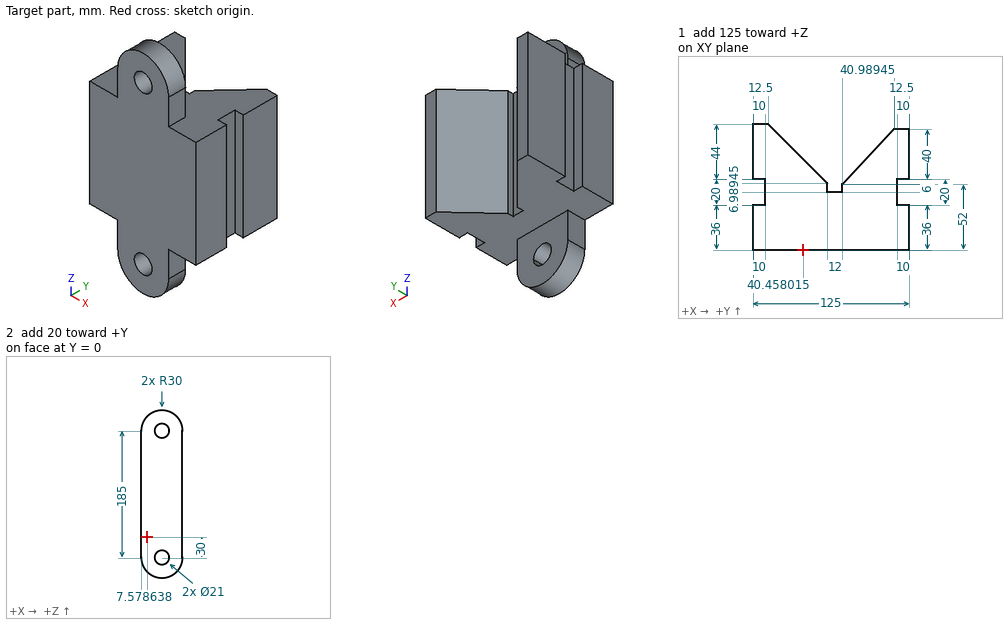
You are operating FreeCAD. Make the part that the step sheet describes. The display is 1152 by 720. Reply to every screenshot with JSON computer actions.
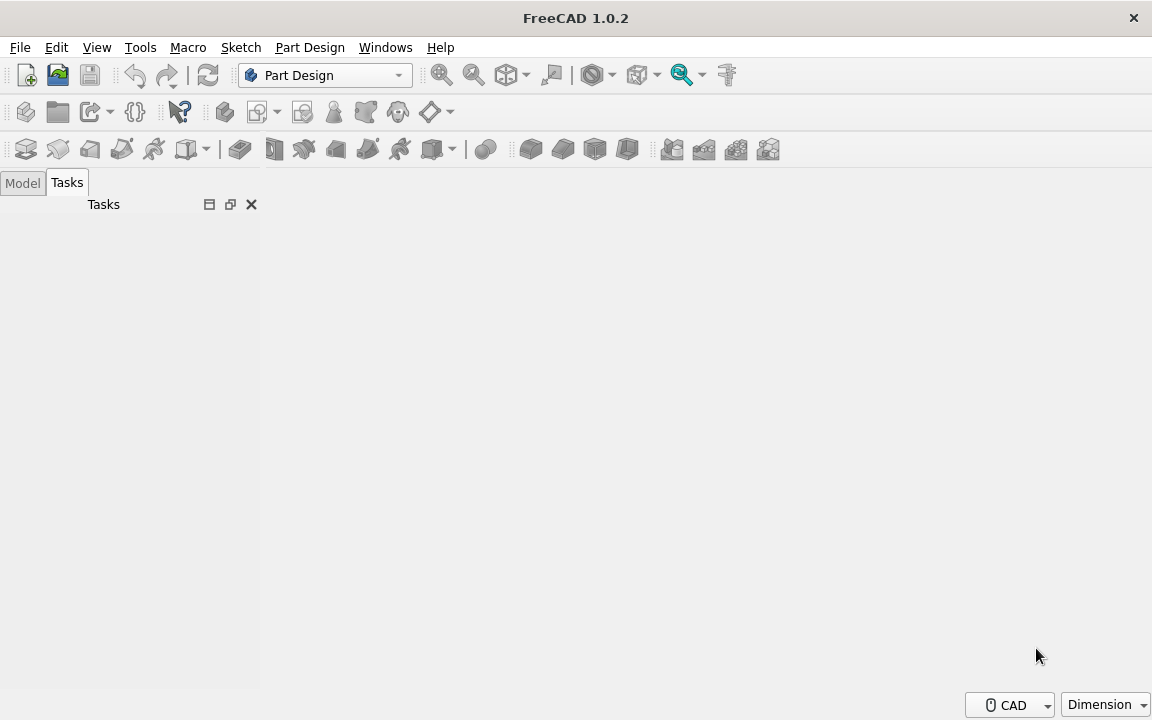
{"action": "key", "text": "ctrl+n"}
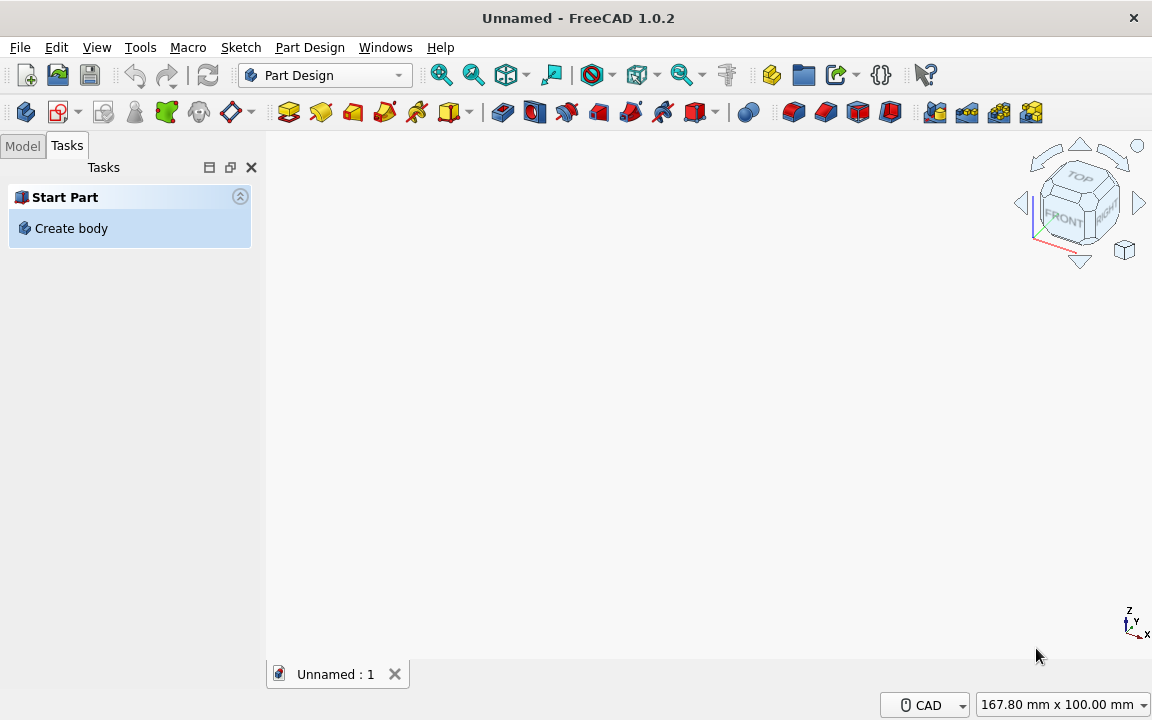
{"action": "left_click", "coordinate": [58, 112]}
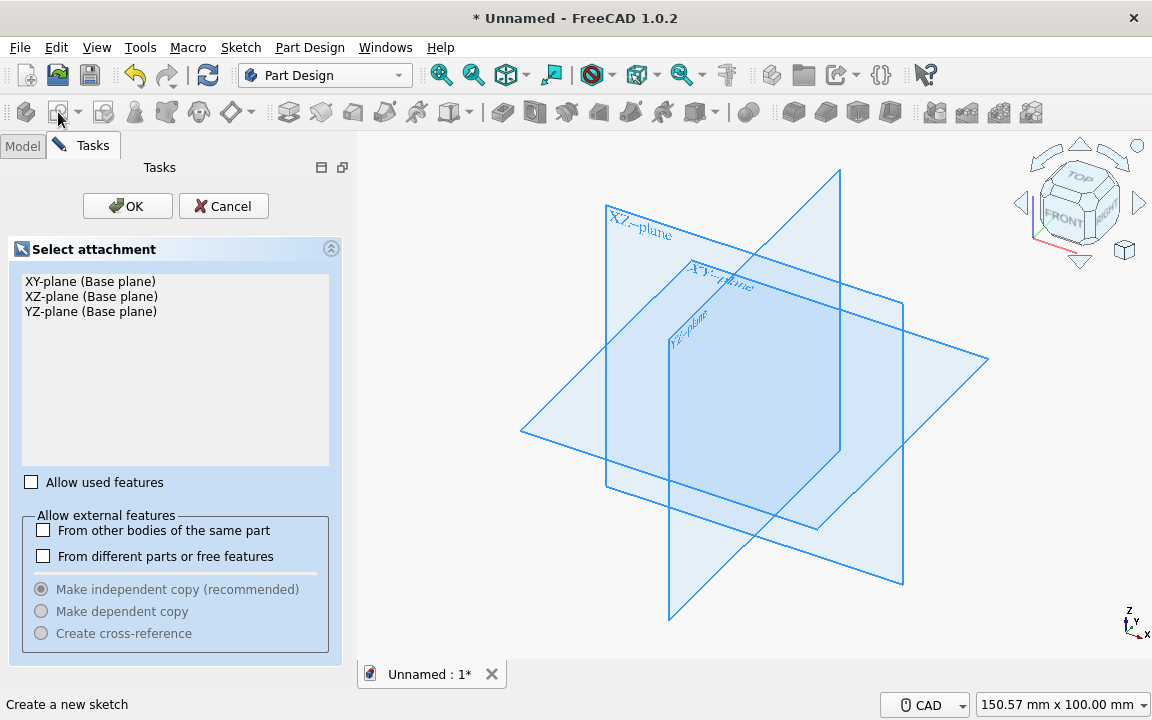
{"action": "left_click", "coordinate": [82, 282]}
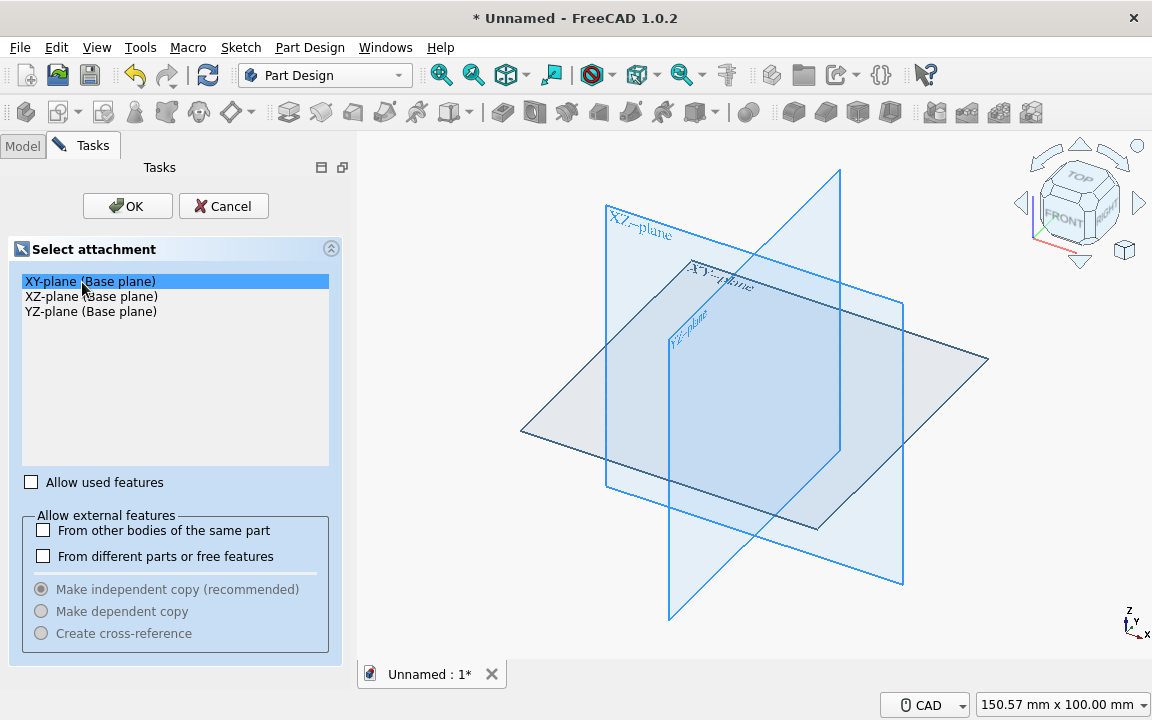
{"action": "left_click", "coordinate": [128, 206]}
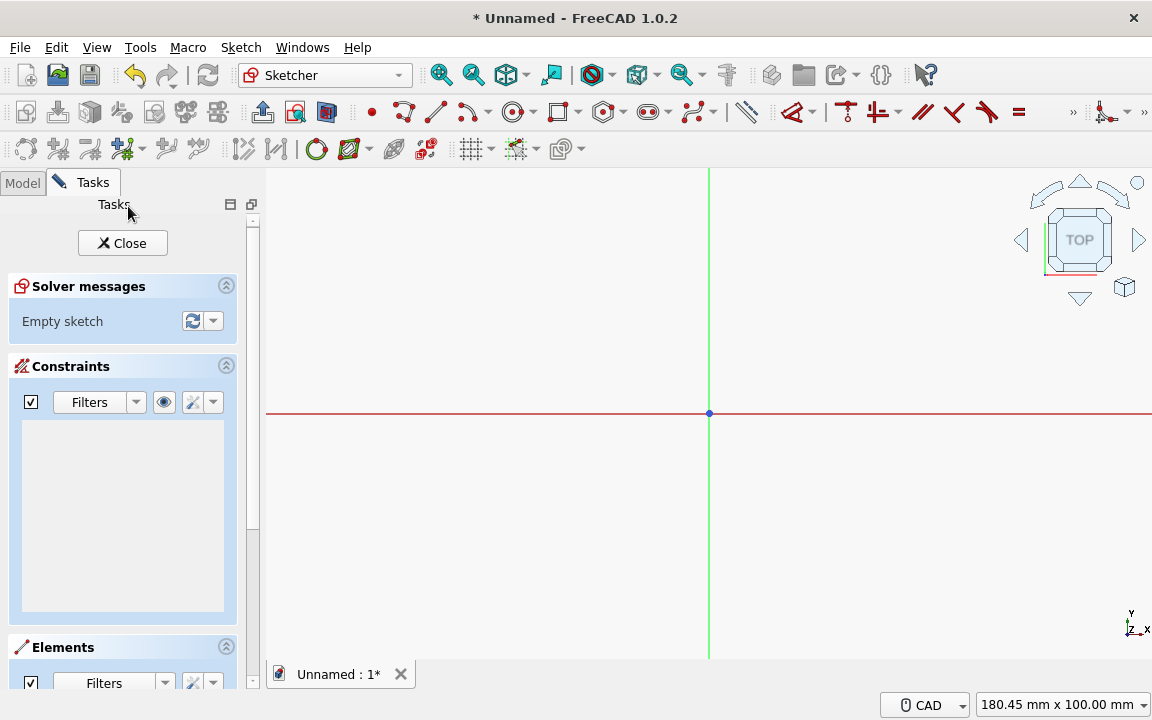
{"action": "scroll", "coordinate": [426, 631], "scroll_direction": "down", "scroll_amount": 3}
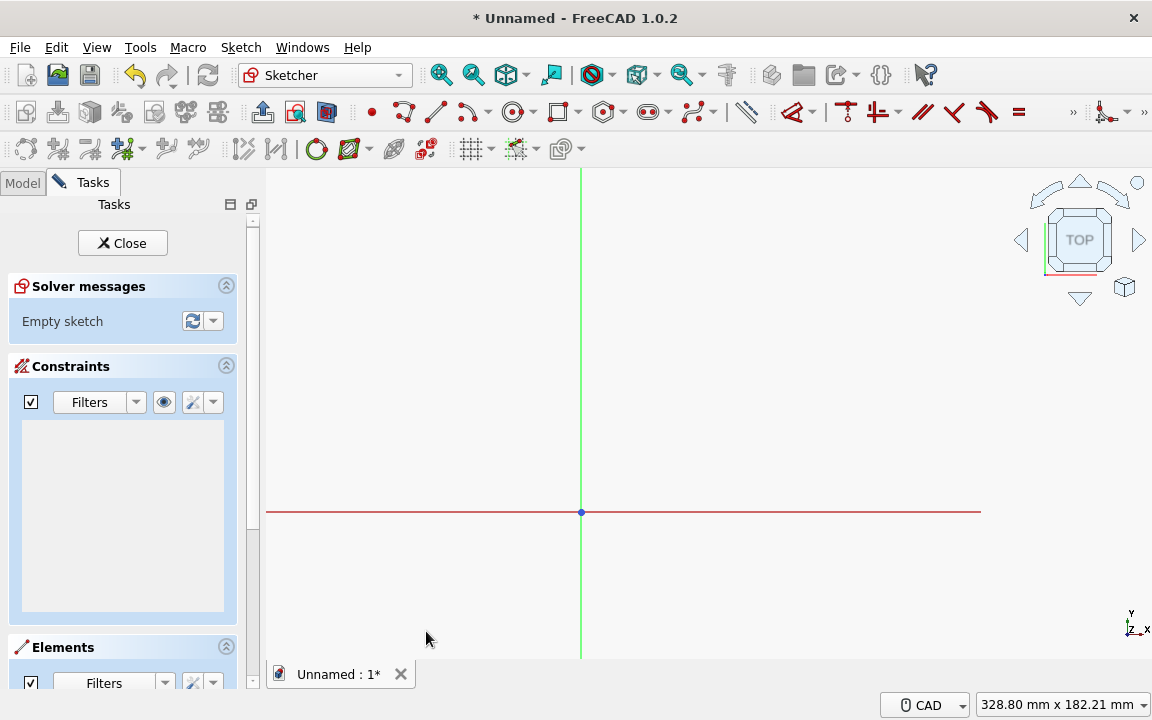
{"action": "key", "text": "g m"}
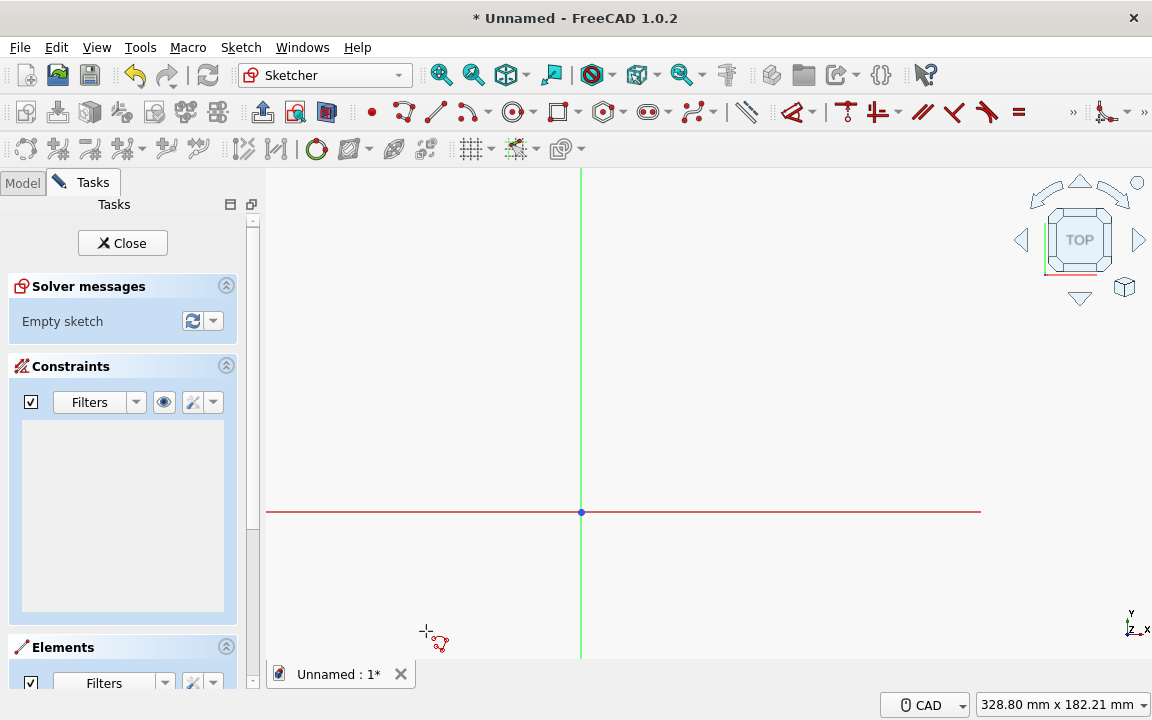
{"action": "left_click", "coordinate": [472, 512]}
{"action": "left_click", "coordinate": [809, 503]}
{"action": "left_click", "coordinate": [809, 415]}
{"action": "left_click", "coordinate": [782, 415]}
{"action": "left_click", "coordinate": [782, 361]}
{"action": "left_click", "coordinate": [809, 361]}
{"action": "left_click", "coordinate": [809, 253]}
{"action": "left_click", "coordinate": [776, 253]}
{"action": "left_click", "coordinate": [665, 372]}
{"action": "left_click", "coordinate": [665, 388]}
{"action": "left_click", "coordinate": [633, 388]}
{"action": "left_click", "coordinate": [633, 369]}
{"action": "left_click", "coordinate": [506, 243]}
{"action": "left_click", "coordinate": [472, 243]}
{"action": "left_click", "coordinate": [472, 361]}
{"action": "left_click", "coordinate": [499, 361]}
{"action": "left_click", "coordinate": [499, 415]}
{"action": "left_click", "coordinate": [472, 415]}
{"action": "left_click", "coordinate": [472, 512]}
{"action": "key", "text": "Escape"}
{"action": "key", "text": "Escape"}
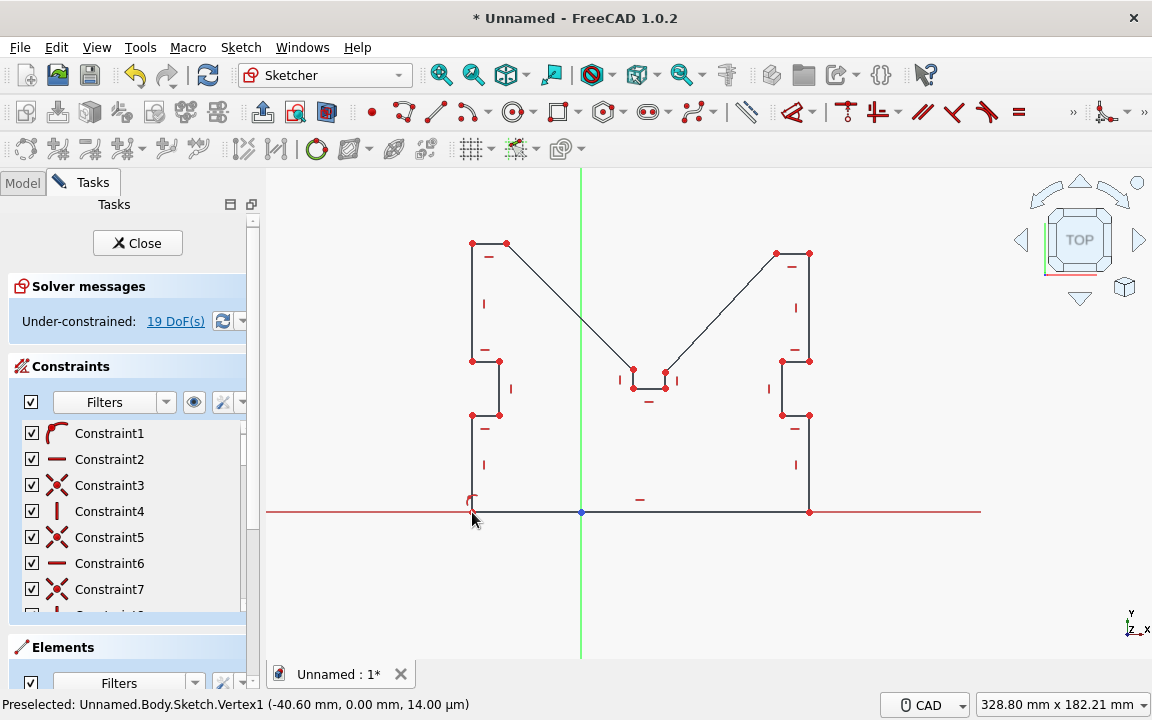
{"action": "key", "text": "d"}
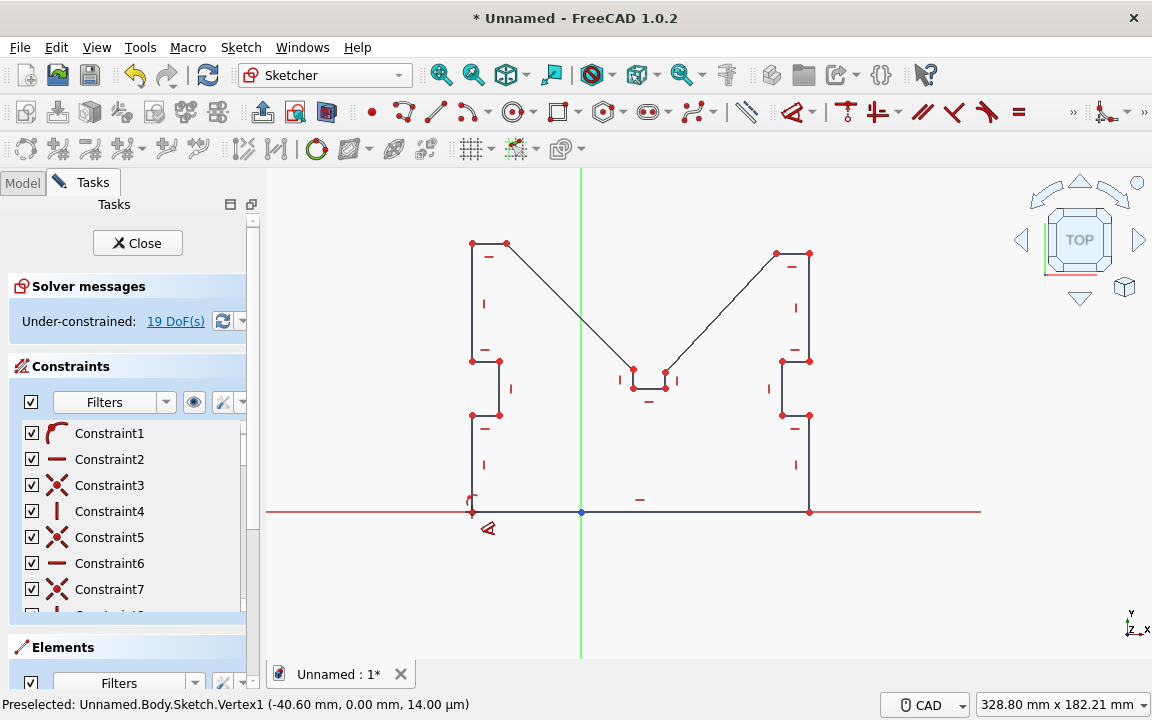
{"action": "scroll", "coordinate": [665, 381], "scroll_direction": "up", "scroll_amount": 5}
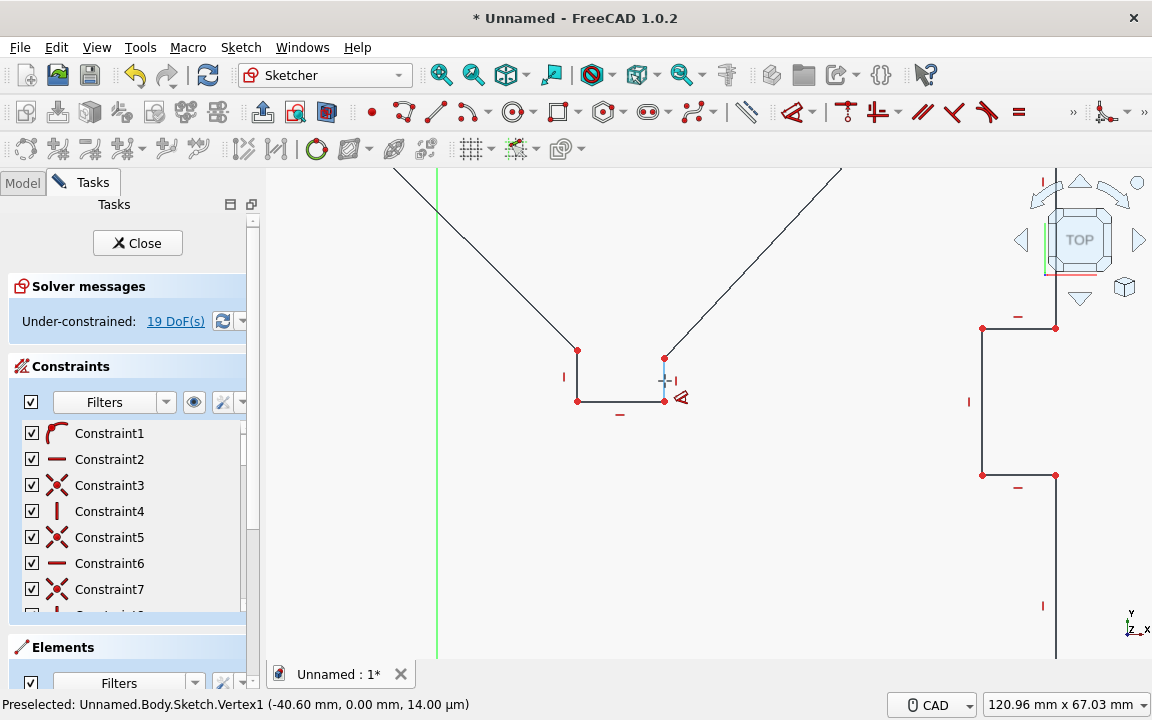
{"action": "left_click", "coordinate": [664, 380]}
{"action": "left_click", "coordinate": [698, 380]}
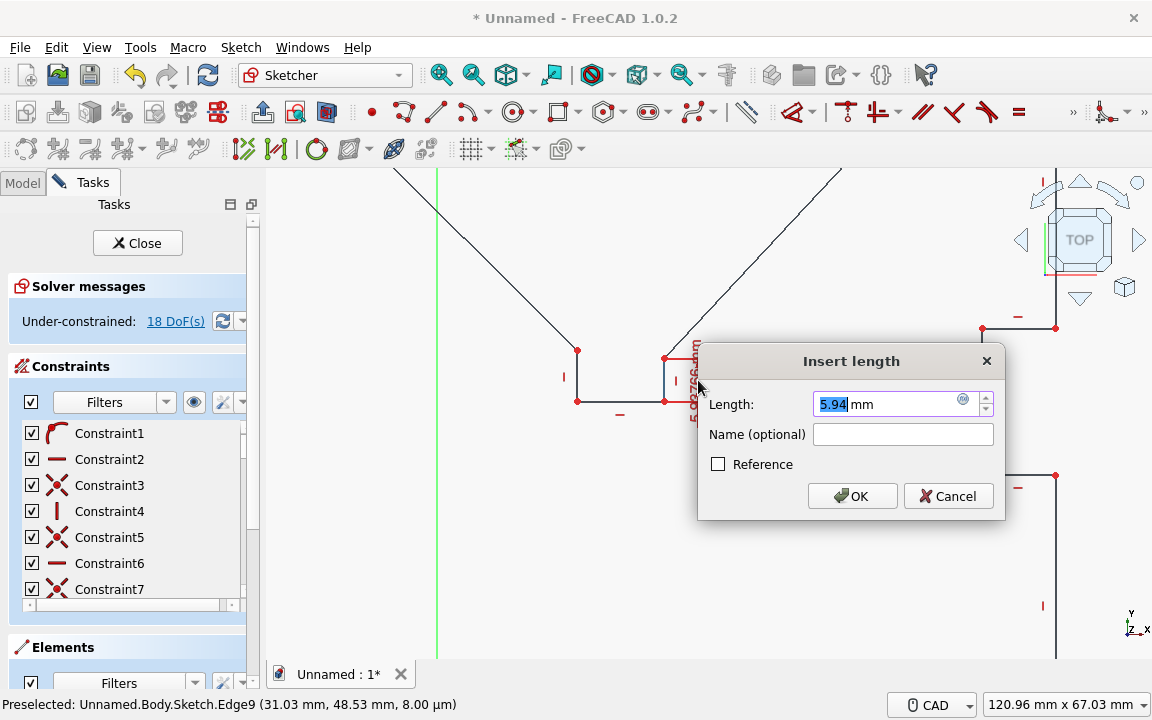
{"action": "type", "text": "6"}
{"action": "key", "text": "Return"}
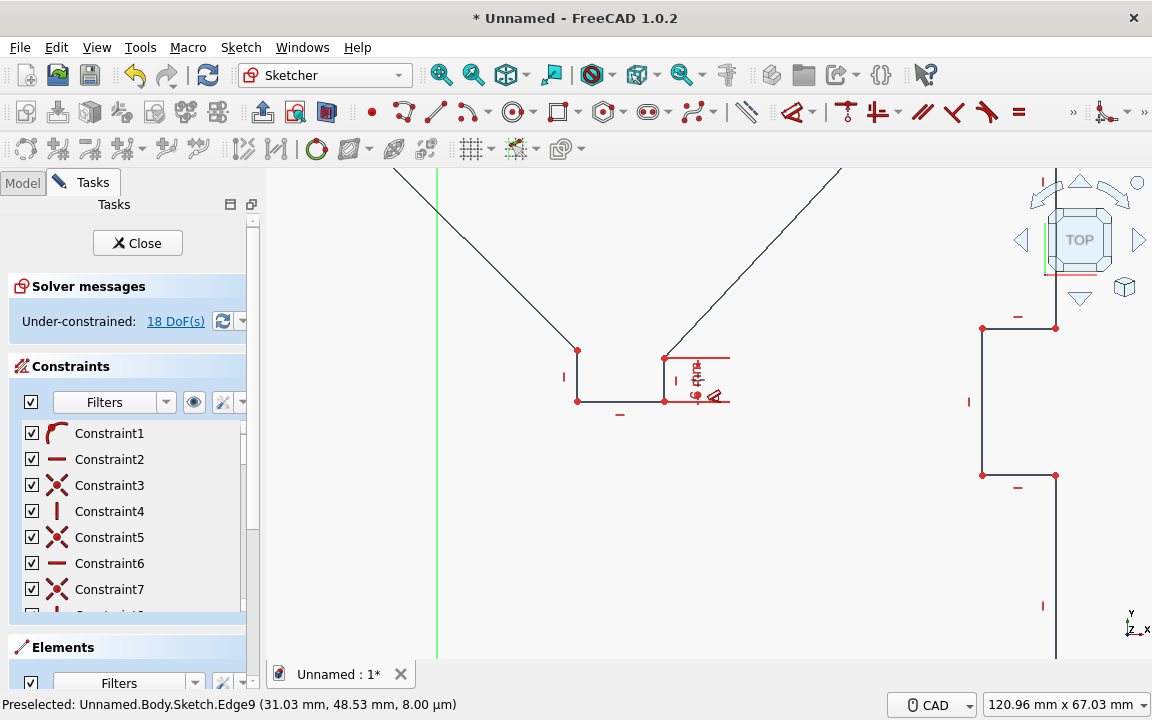
{"action": "scroll", "coordinate": [675, 449], "scroll_direction": "down", "scroll_amount": 4}